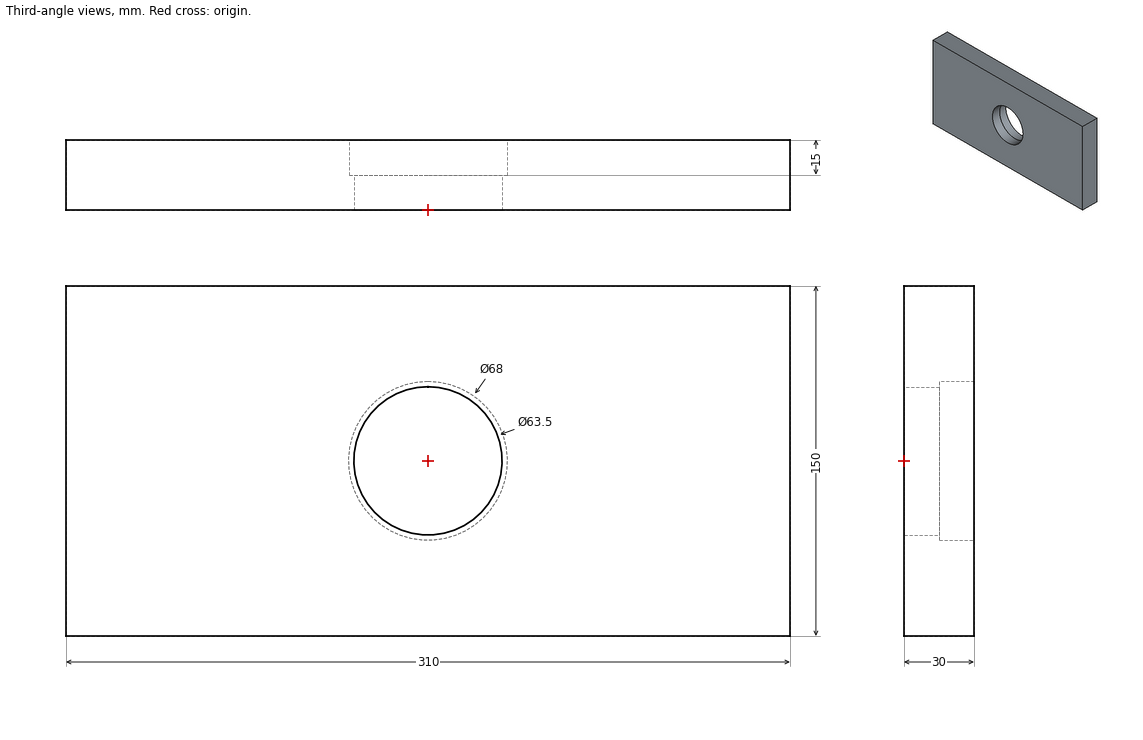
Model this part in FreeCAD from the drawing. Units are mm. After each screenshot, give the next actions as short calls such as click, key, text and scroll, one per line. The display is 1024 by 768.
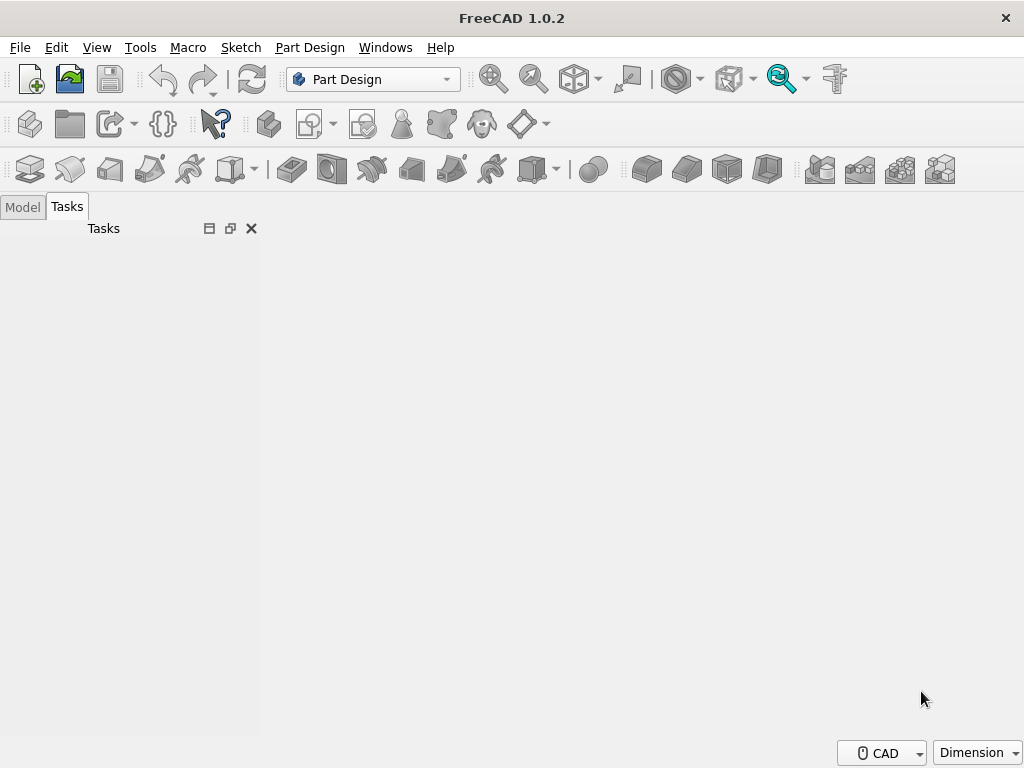
click(30, 80)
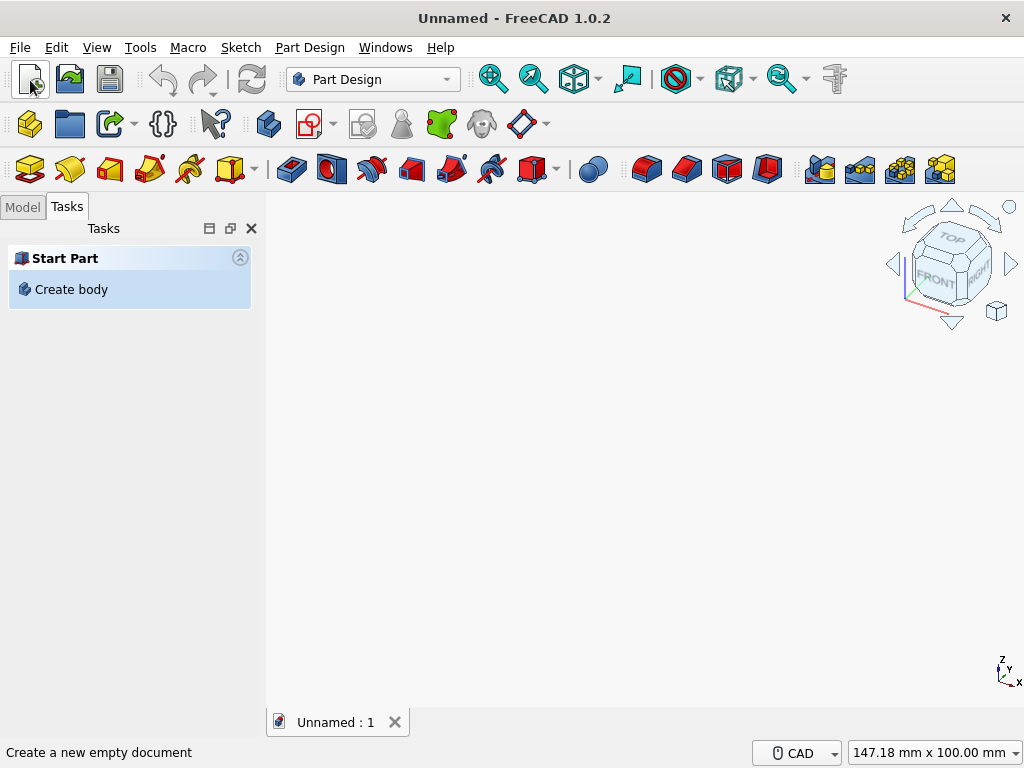
click(310, 124)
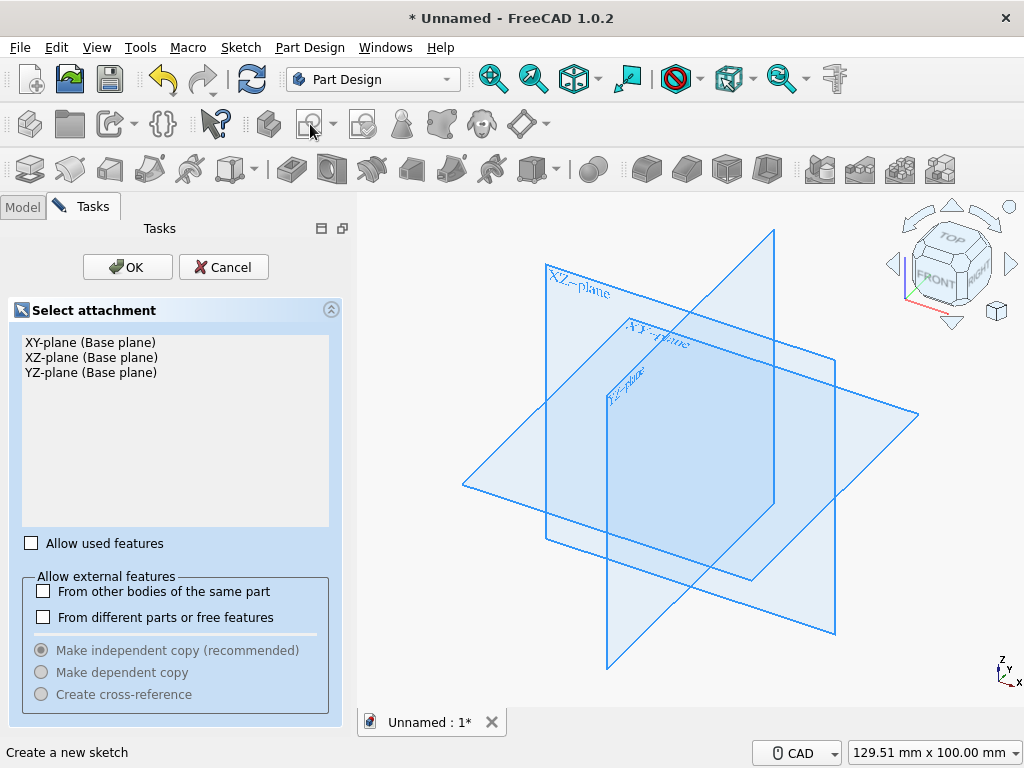
click(82, 358)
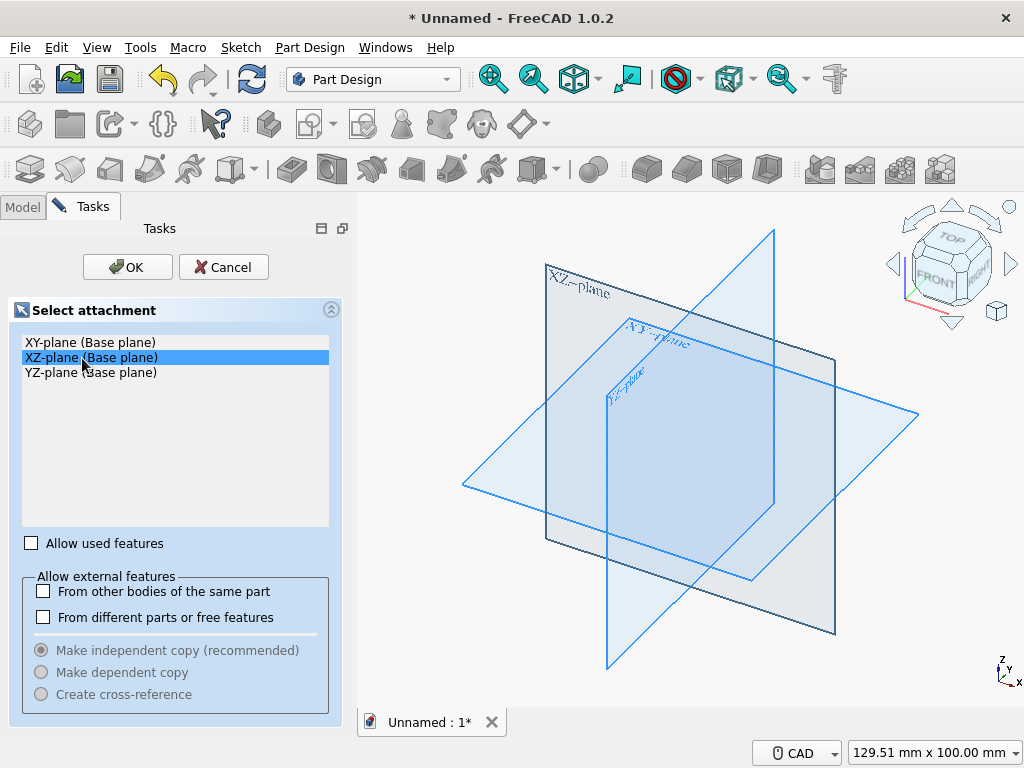
click(128, 267)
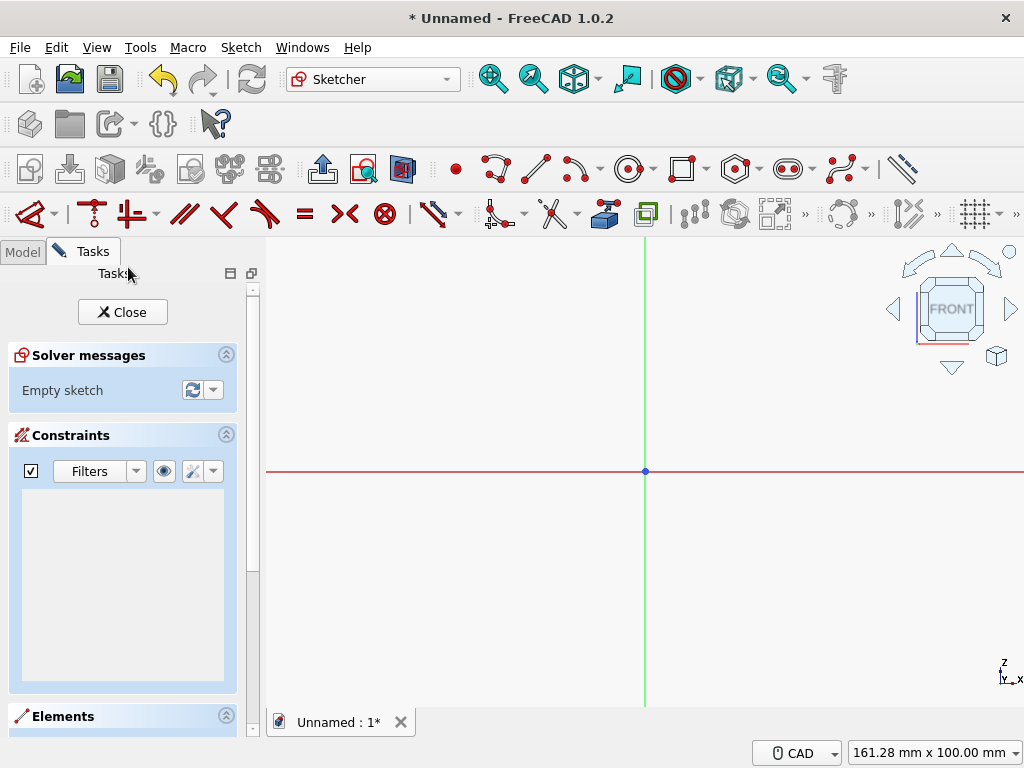
scroll(547, 472, down, 6)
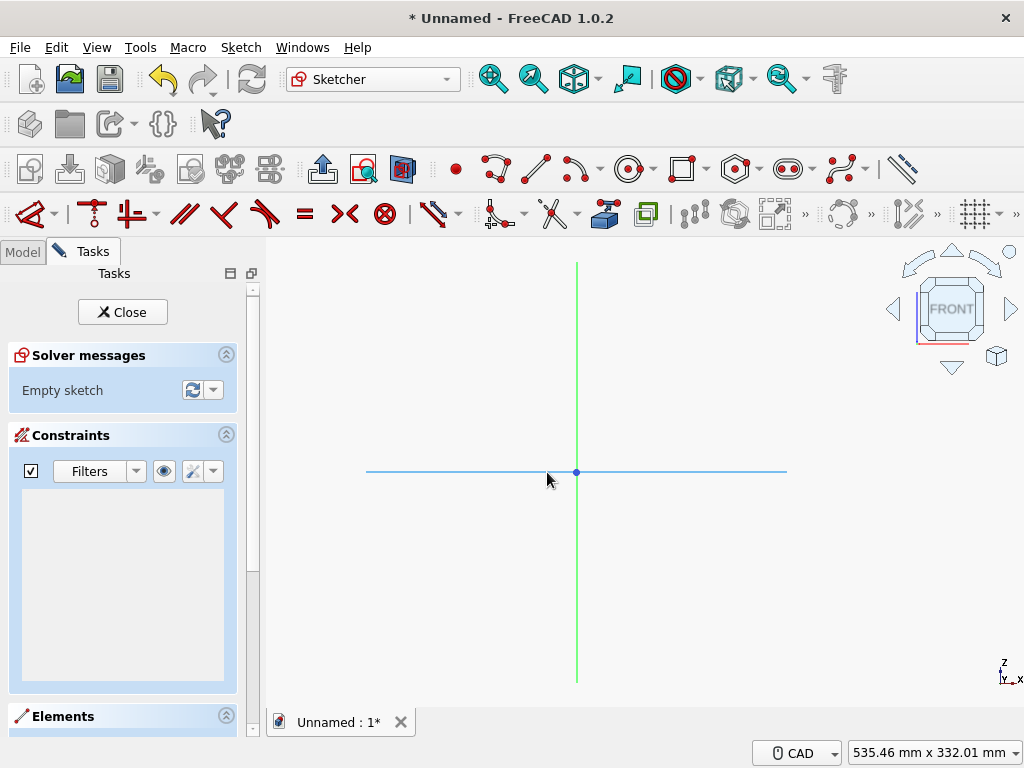
key(g)
key(v)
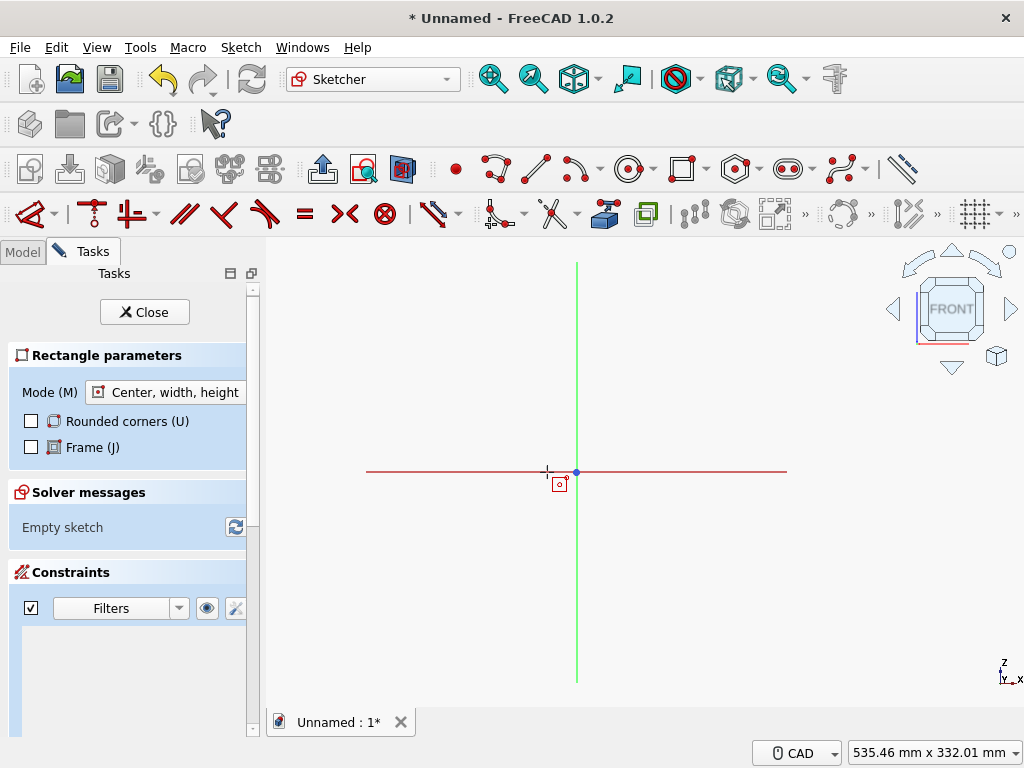
click(577, 472)
move(796, 366)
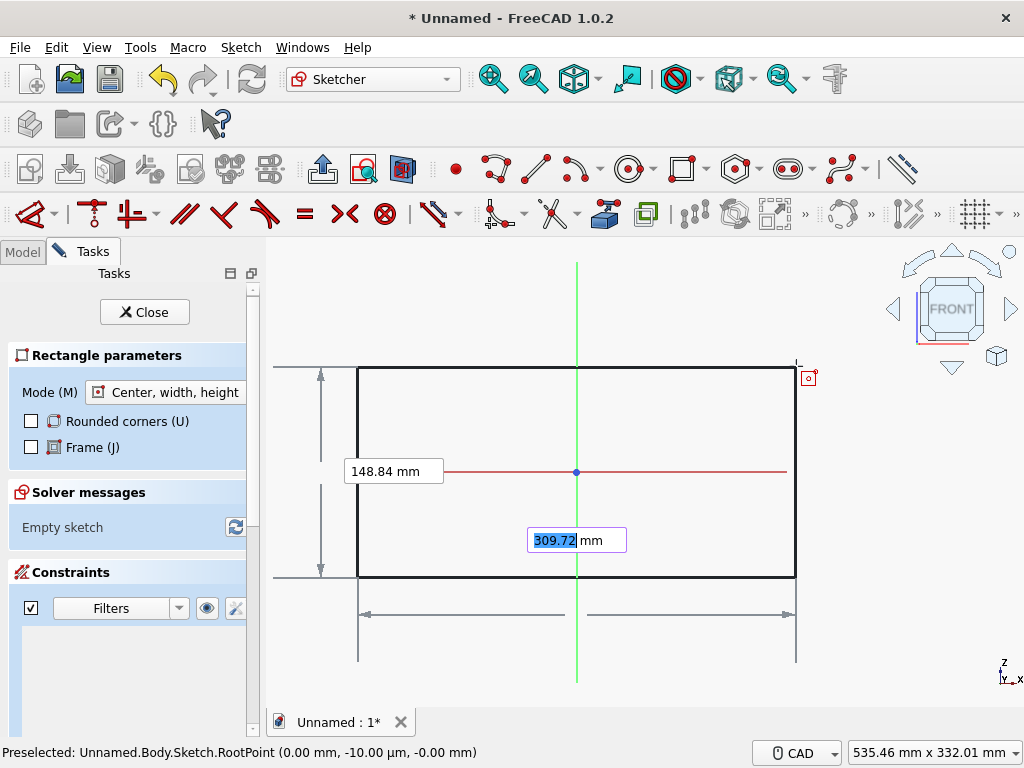
text(310)
key(Tab)
text(150)
key(Return)
key(Escape)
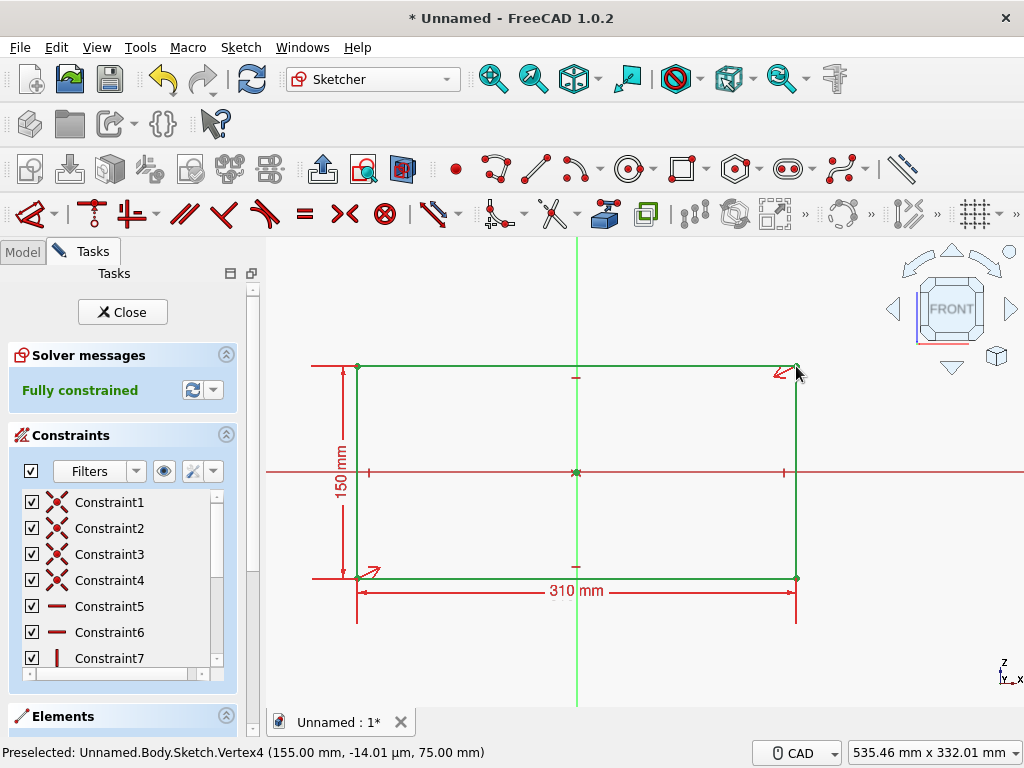
click(123, 312)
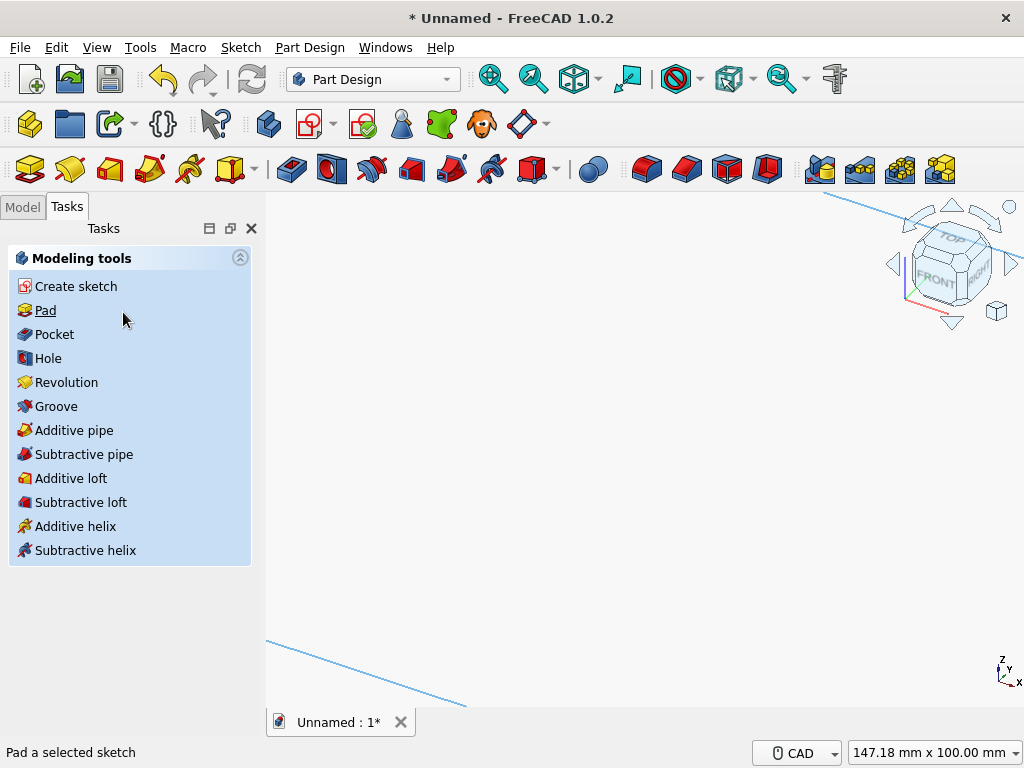
click(30, 170)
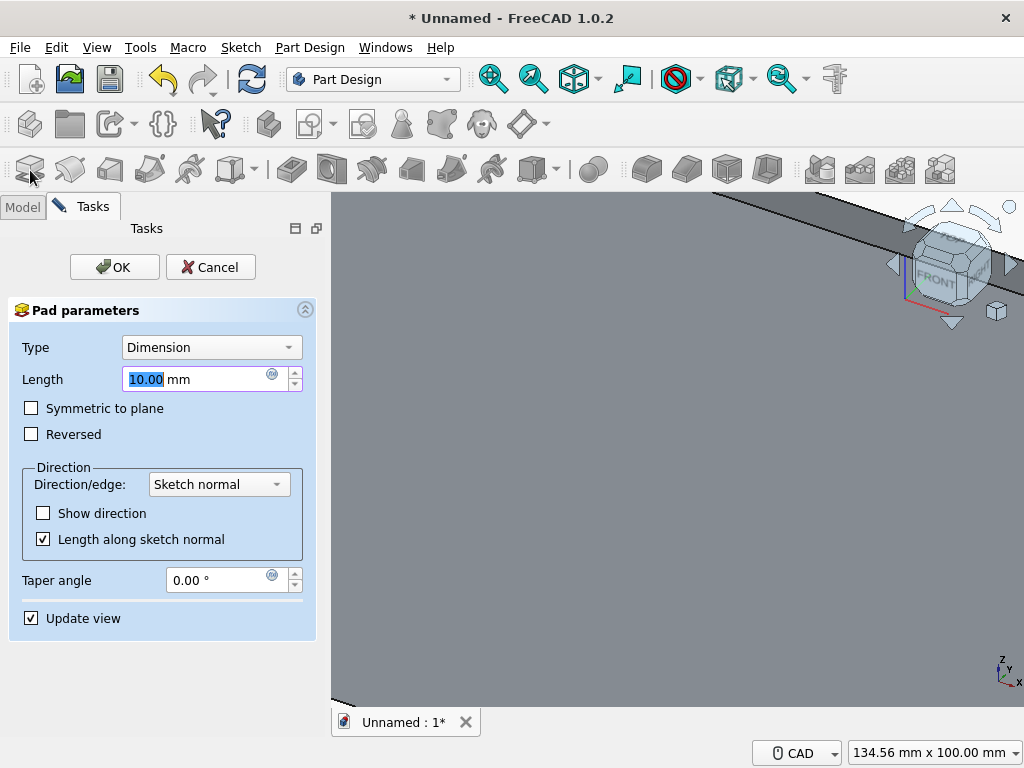
text(30)
key(Tab)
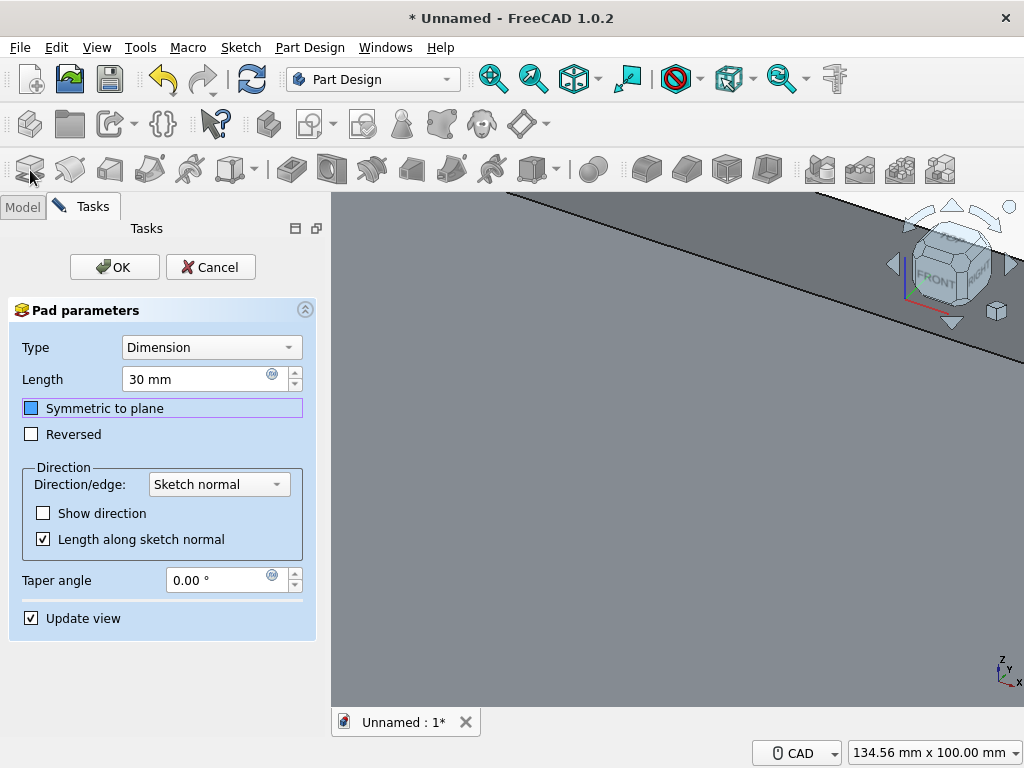
click(30, 434)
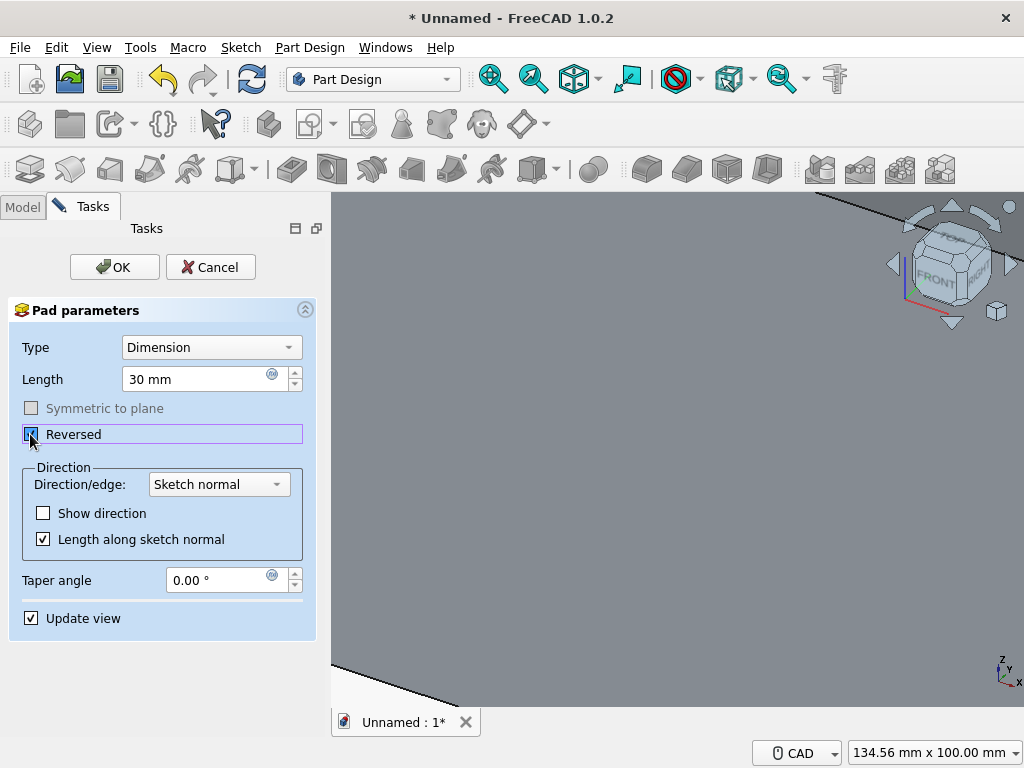
click(115, 267)